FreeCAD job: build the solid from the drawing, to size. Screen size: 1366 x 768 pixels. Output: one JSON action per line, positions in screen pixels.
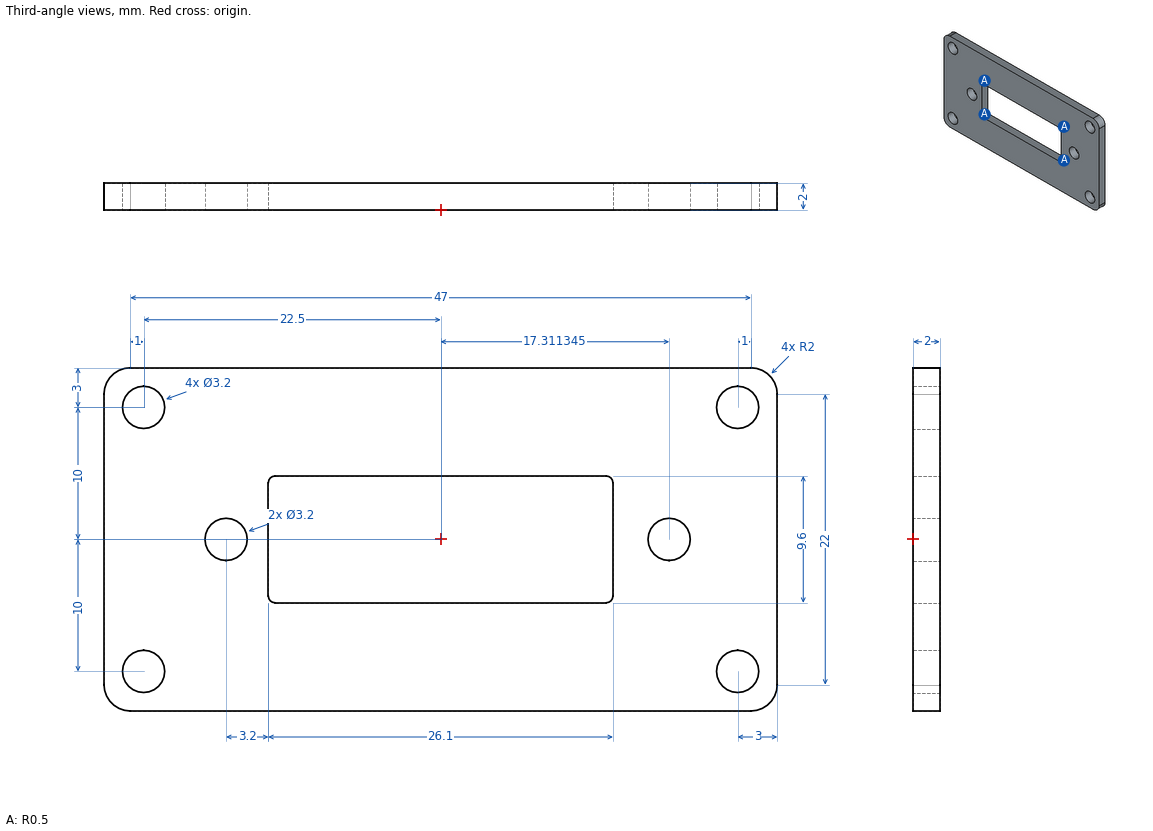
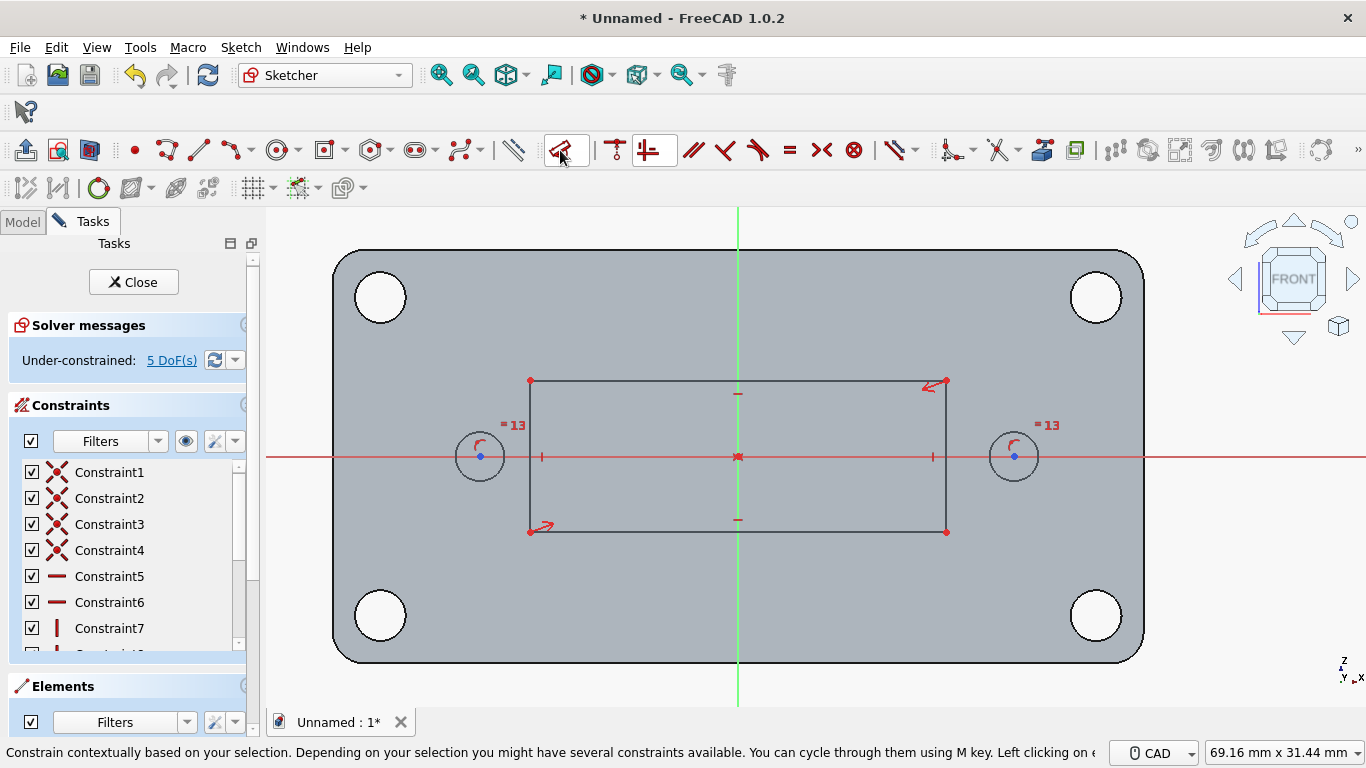
{"action": "left_click", "coordinate": [497, 439]}
{"action": "left_click", "coordinate": [495, 402]}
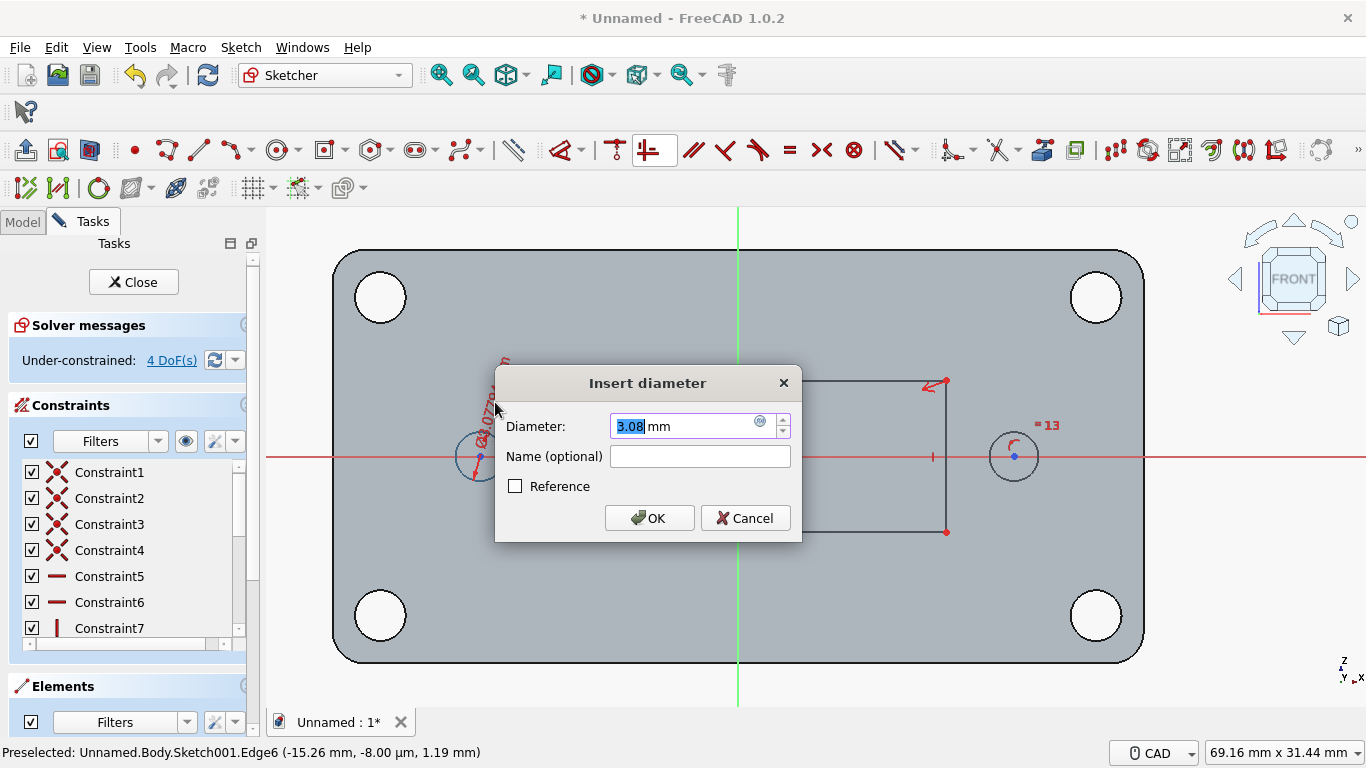
{"action": "type", "text": "3.2"}
{"action": "key", "text": "Return"}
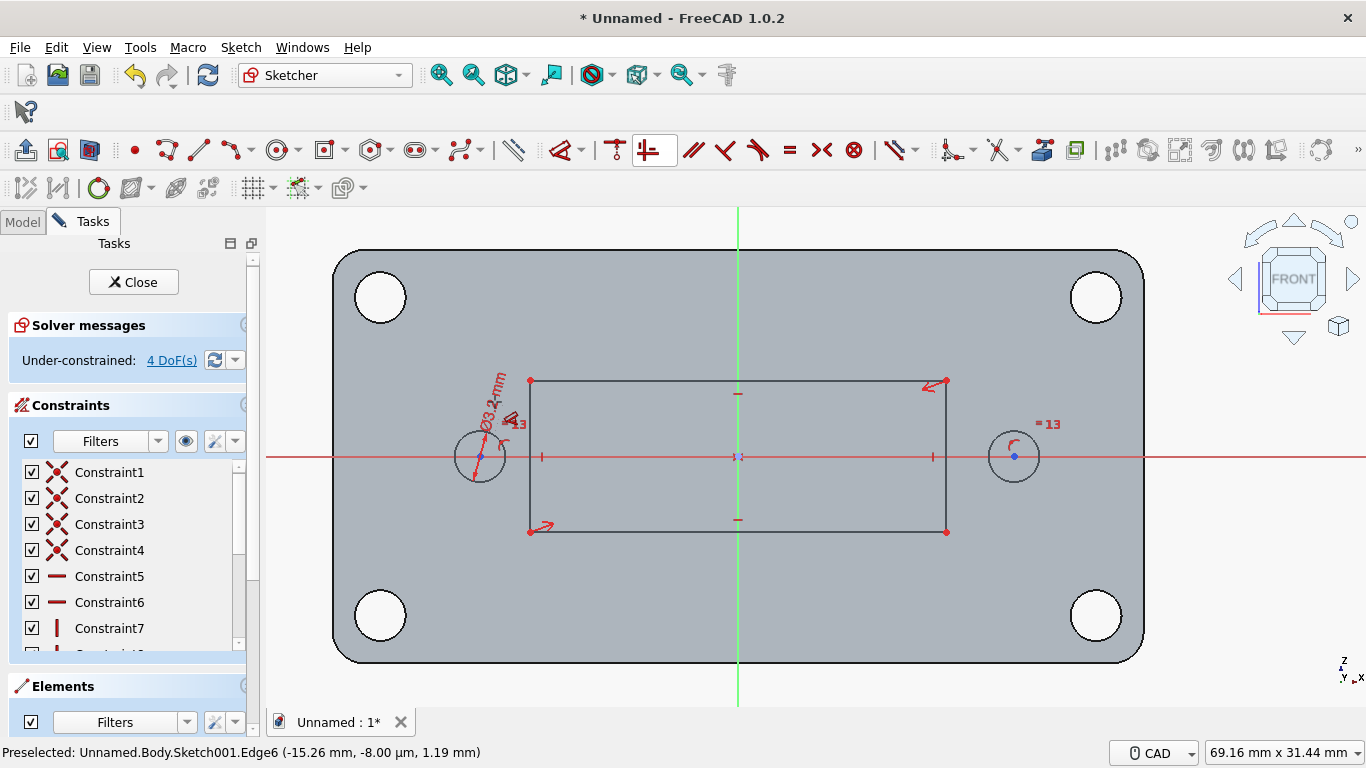
{"action": "left_click", "coordinate": [946, 487]}
{"action": "left_click", "coordinate": [980, 422]}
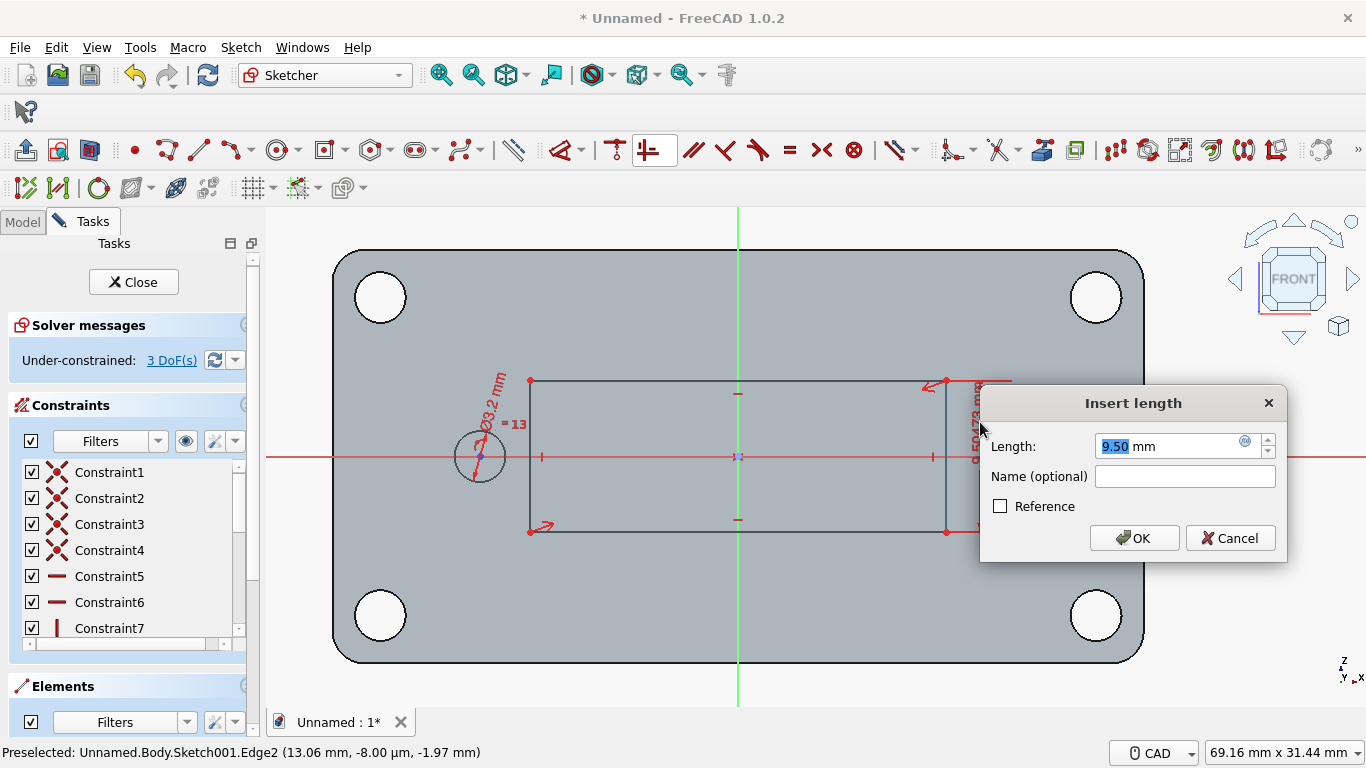
{"action": "type", "text": "9.6"}
{"action": "key", "text": "Return"}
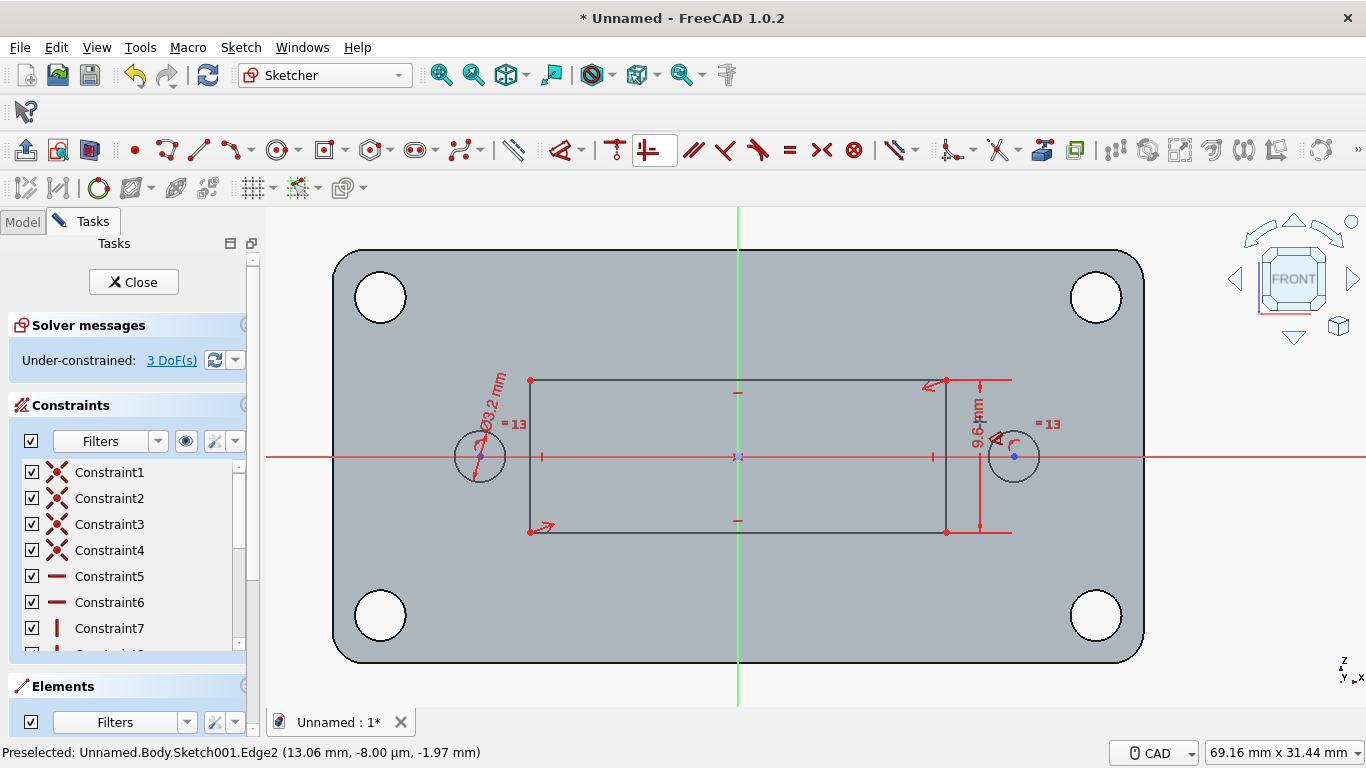
{"action": "left_click", "coordinate": [655, 533]}
{"action": "left_click", "coordinate": [643, 567]}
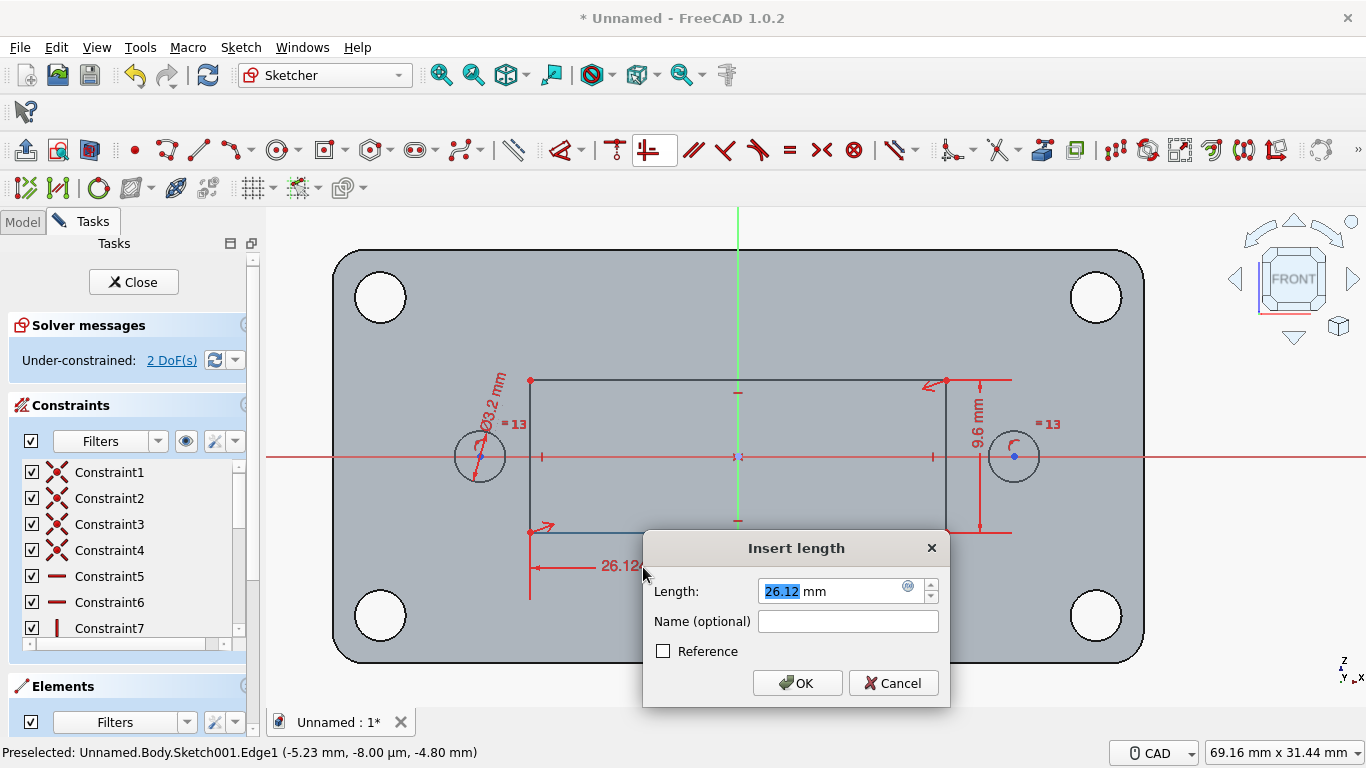
{"action": "type", "text": "26.1"}
{"action": "key", "text": "Return"}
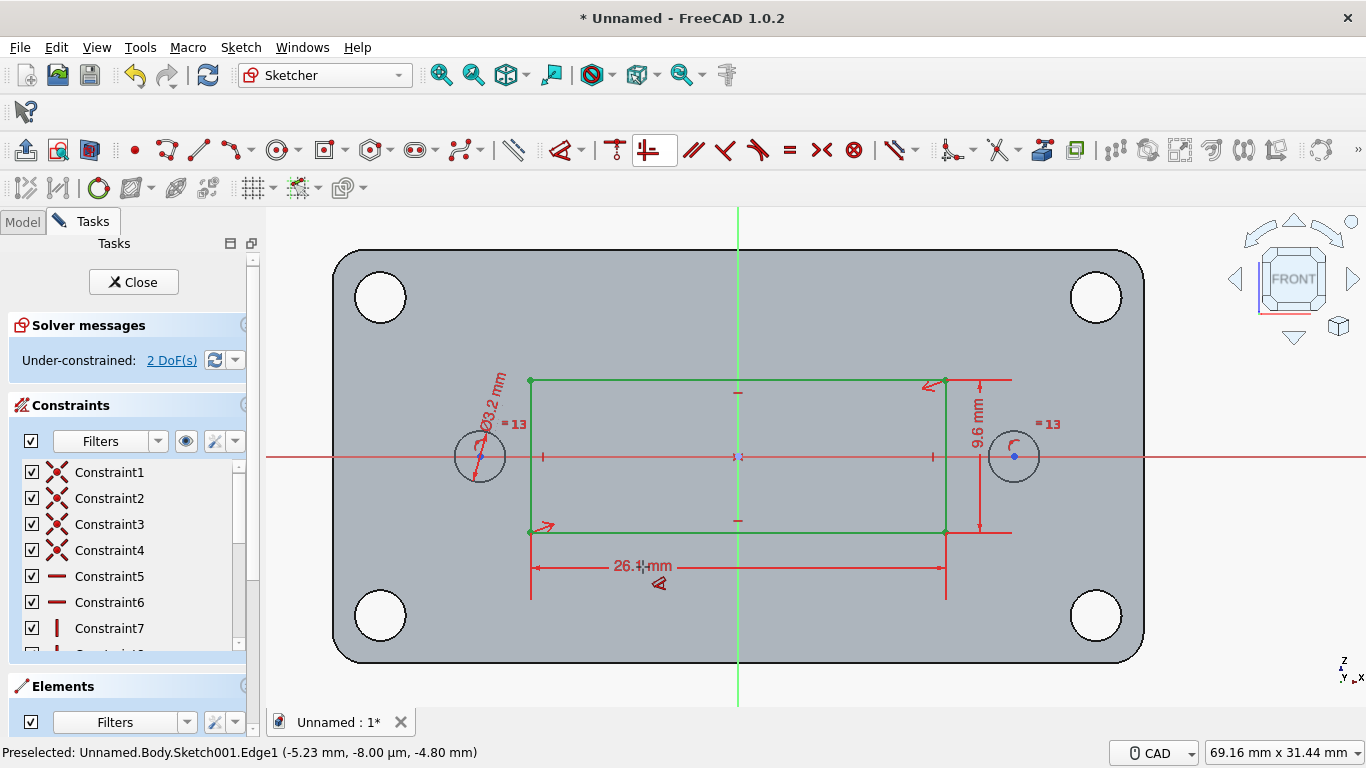
{"action": "left_click", "coordinate": [531, 533]}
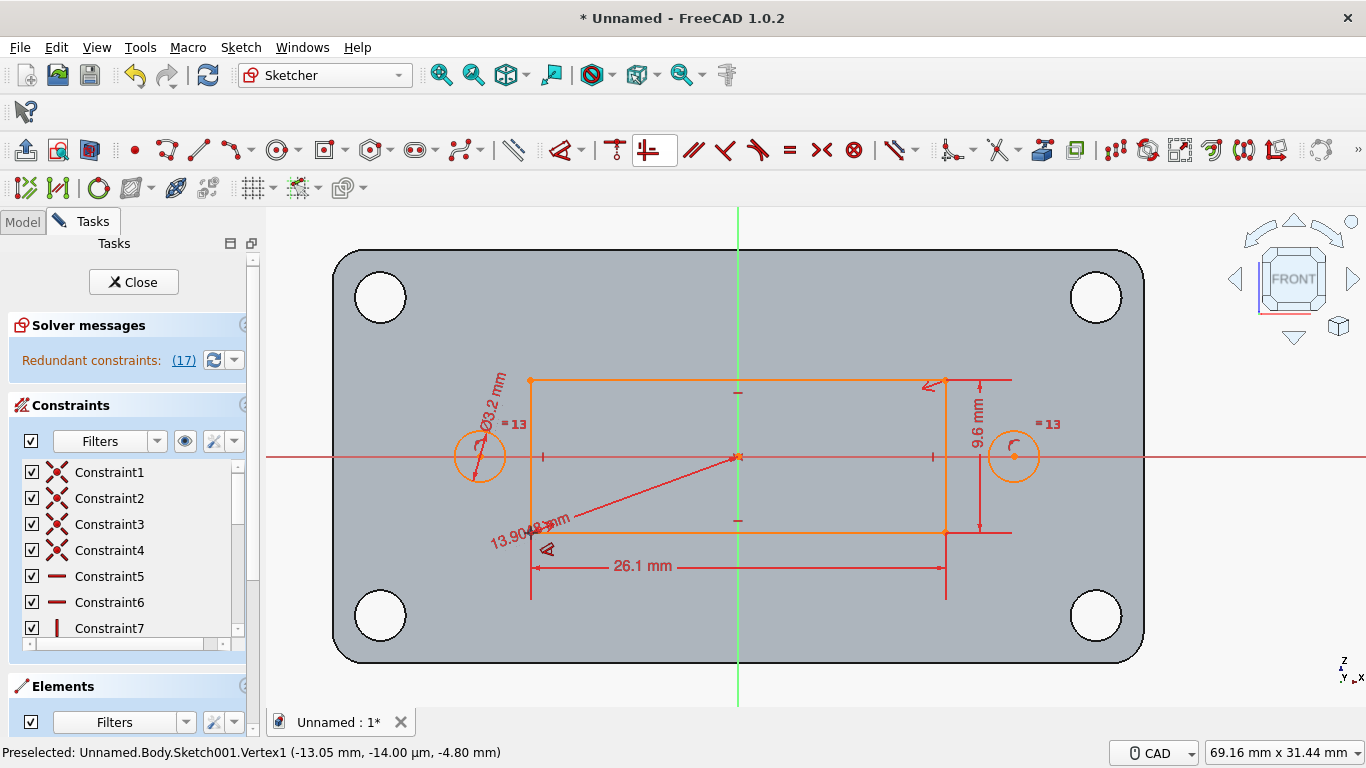
{"action": "left_click", "coordinate": [480, 457]}
{"action": "left_click", "coordinate": [505, 567]}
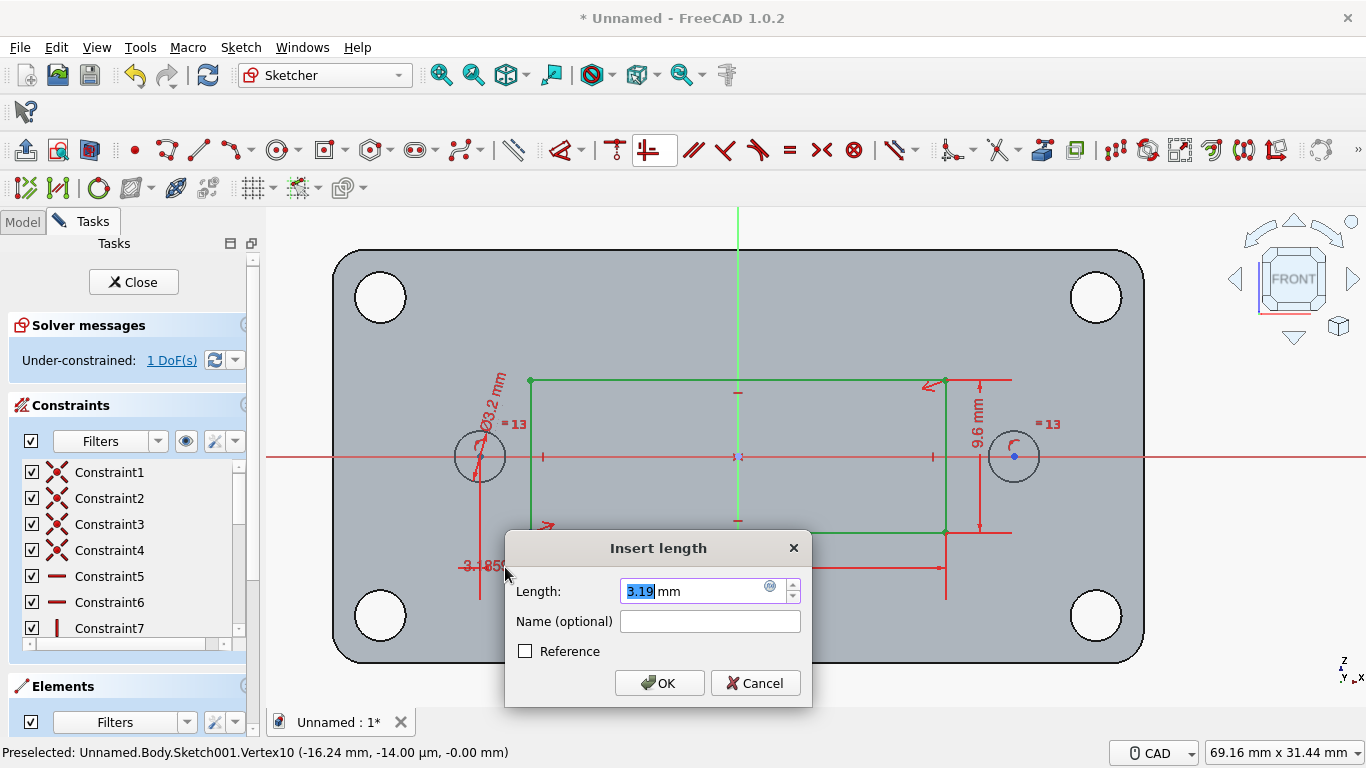
{"action": "type", "text": "3.2"}
{"action": "key", "text": "Return"}